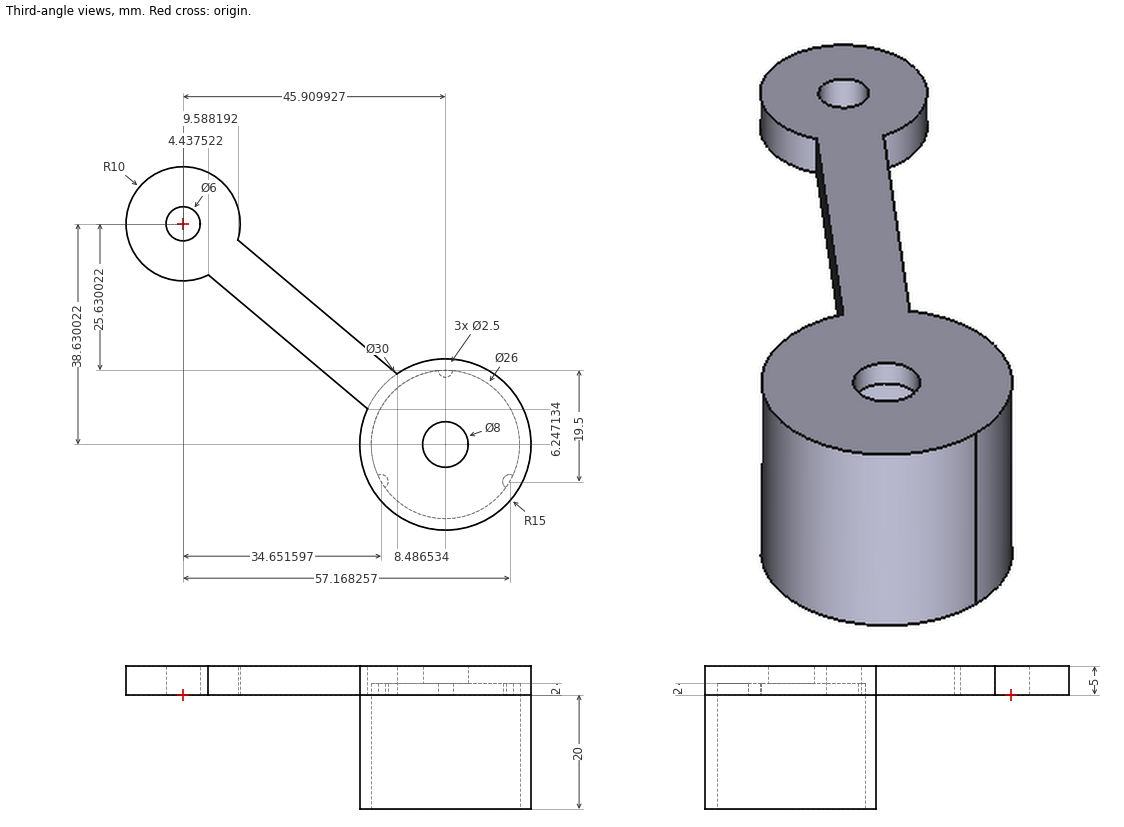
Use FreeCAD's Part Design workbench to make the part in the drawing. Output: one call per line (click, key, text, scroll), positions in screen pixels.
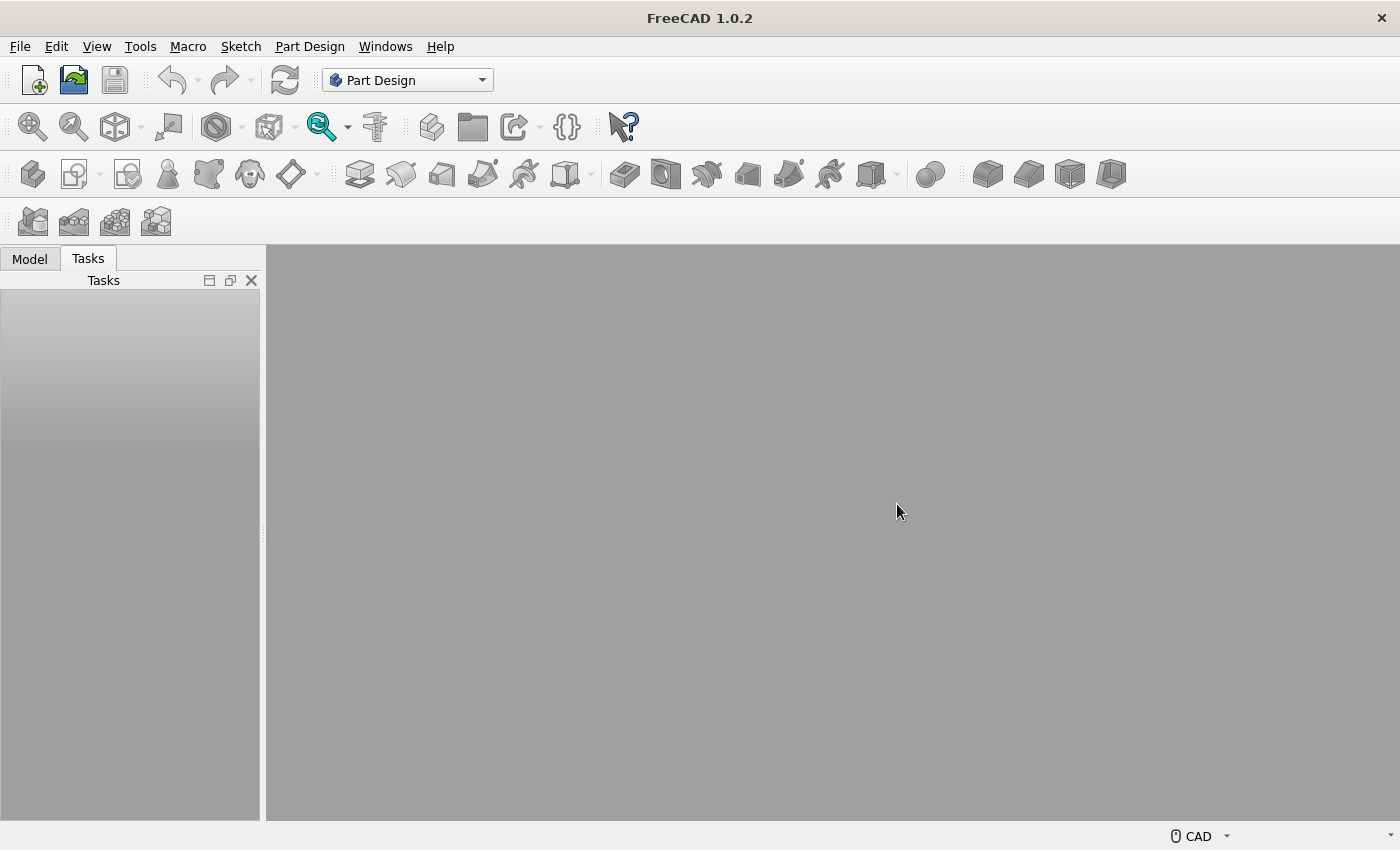
click(33, 80)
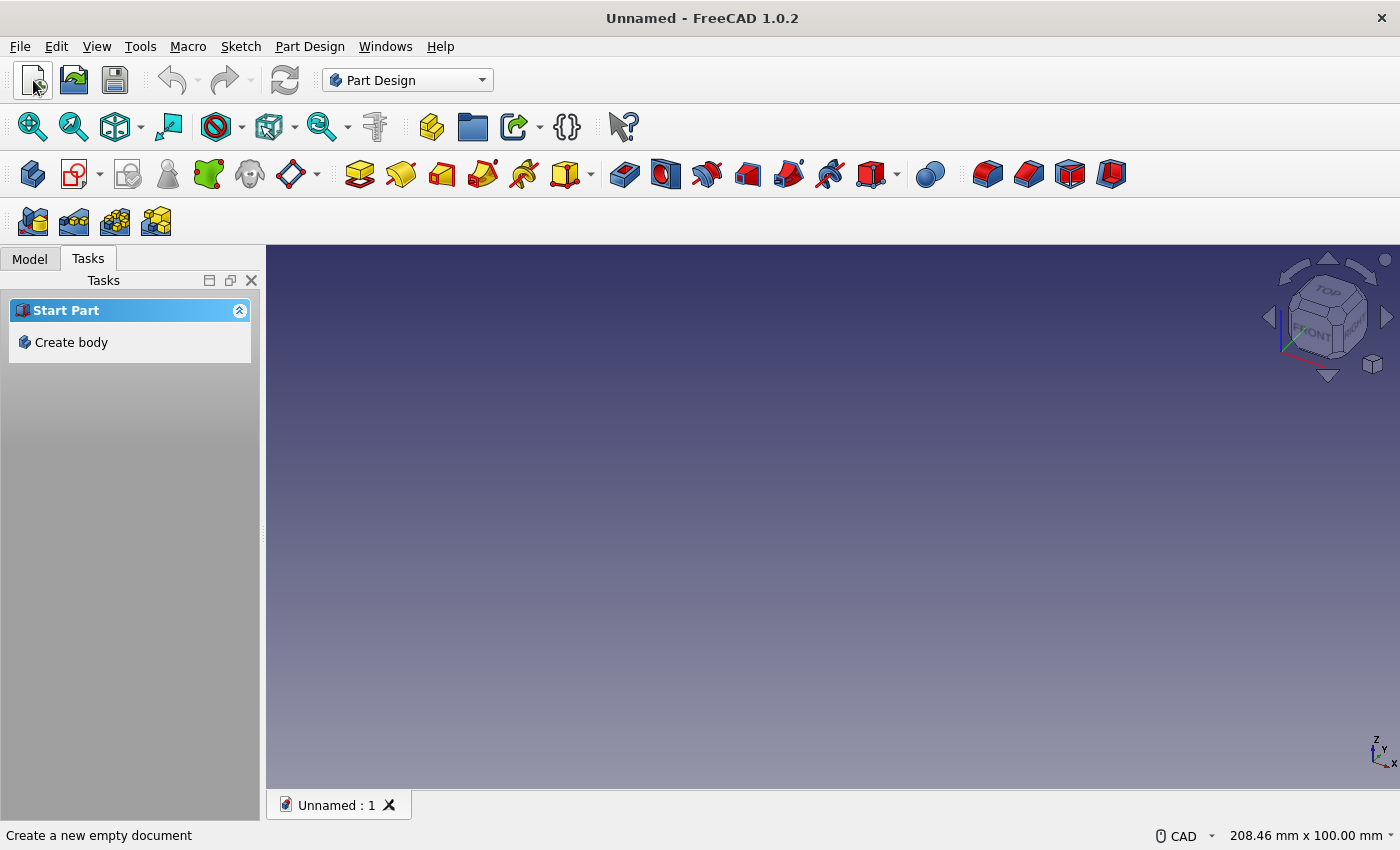
click(74, 174)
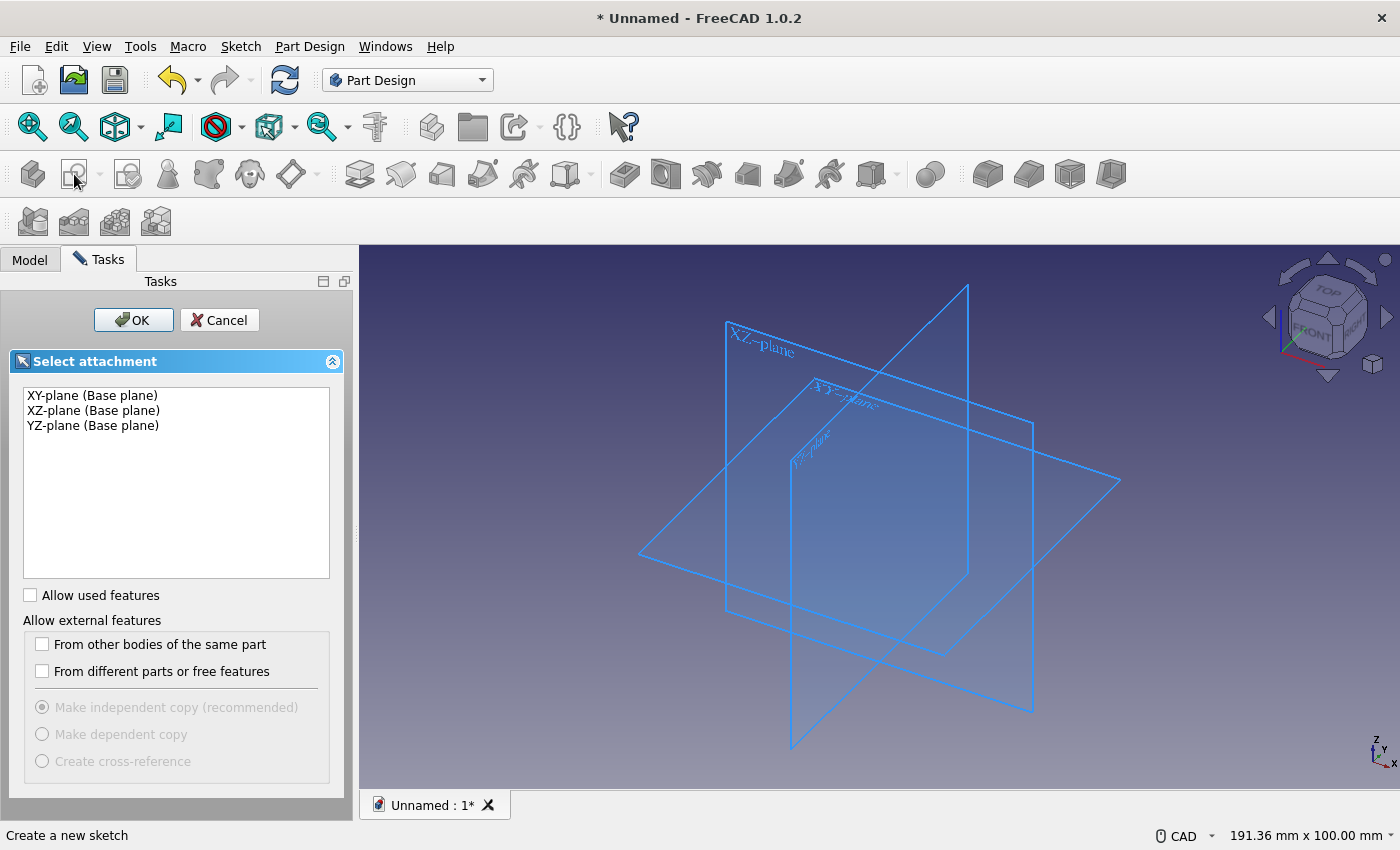
click(84, 396)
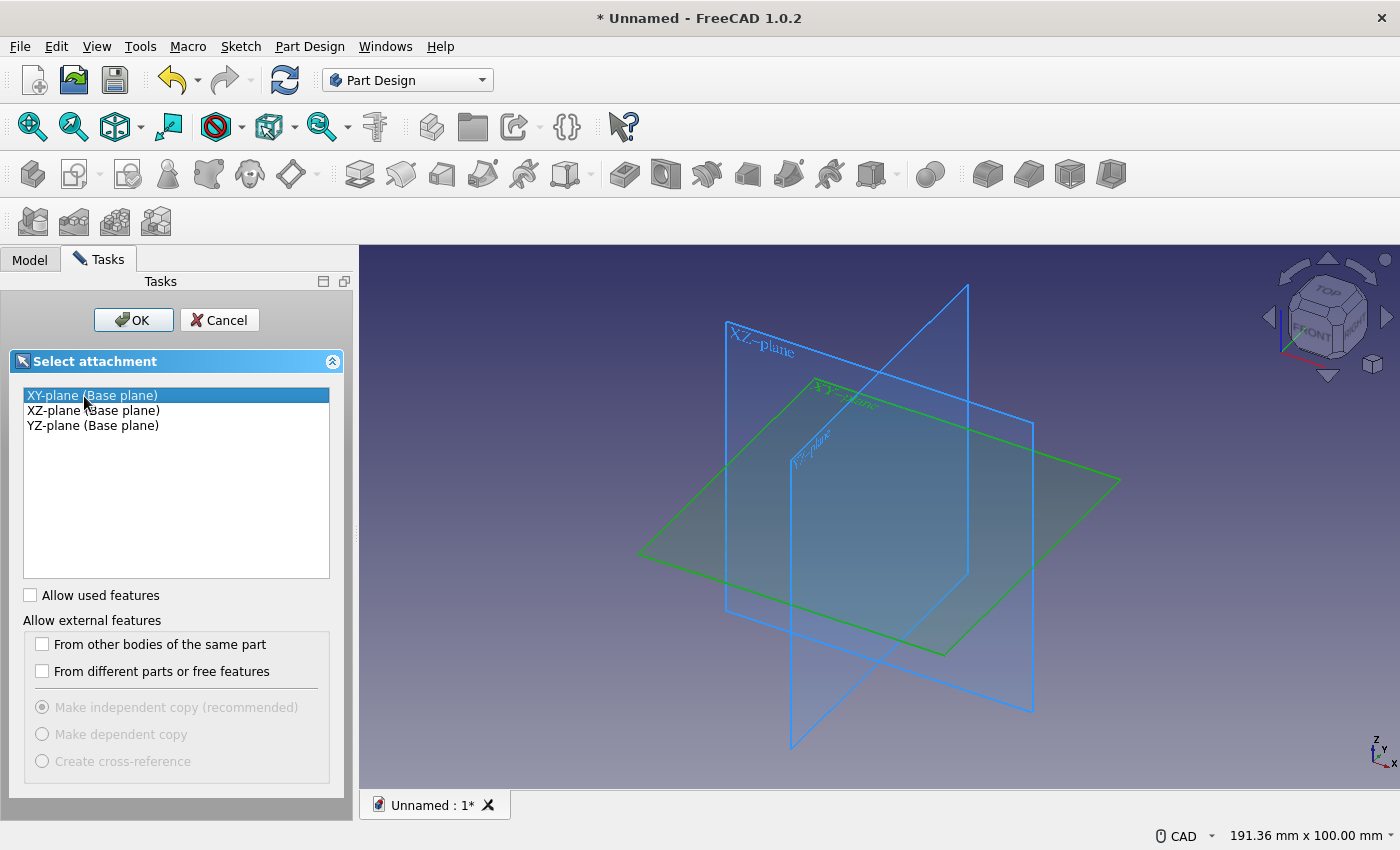
click(134, 320)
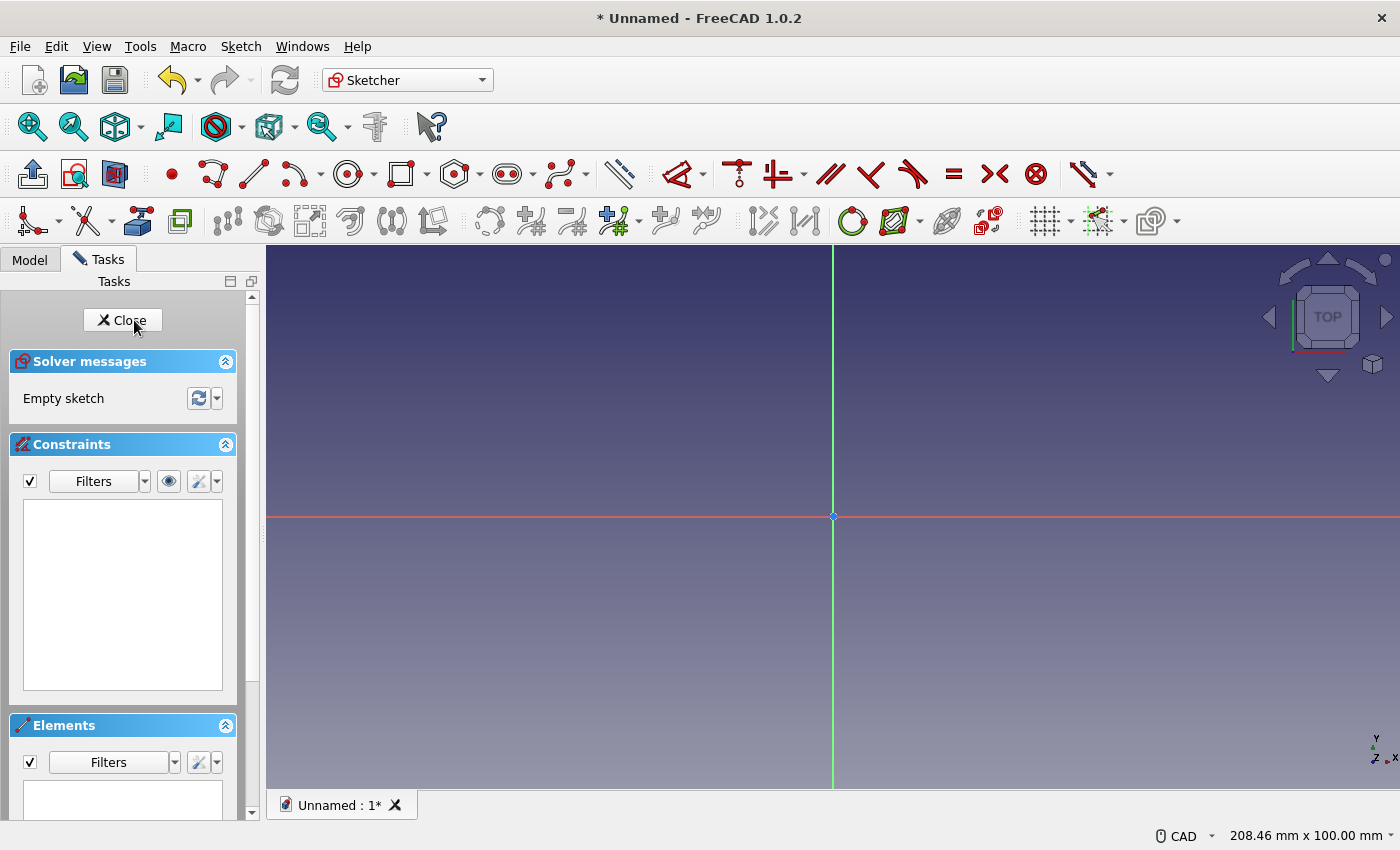
scroll(294, 273, down, 1)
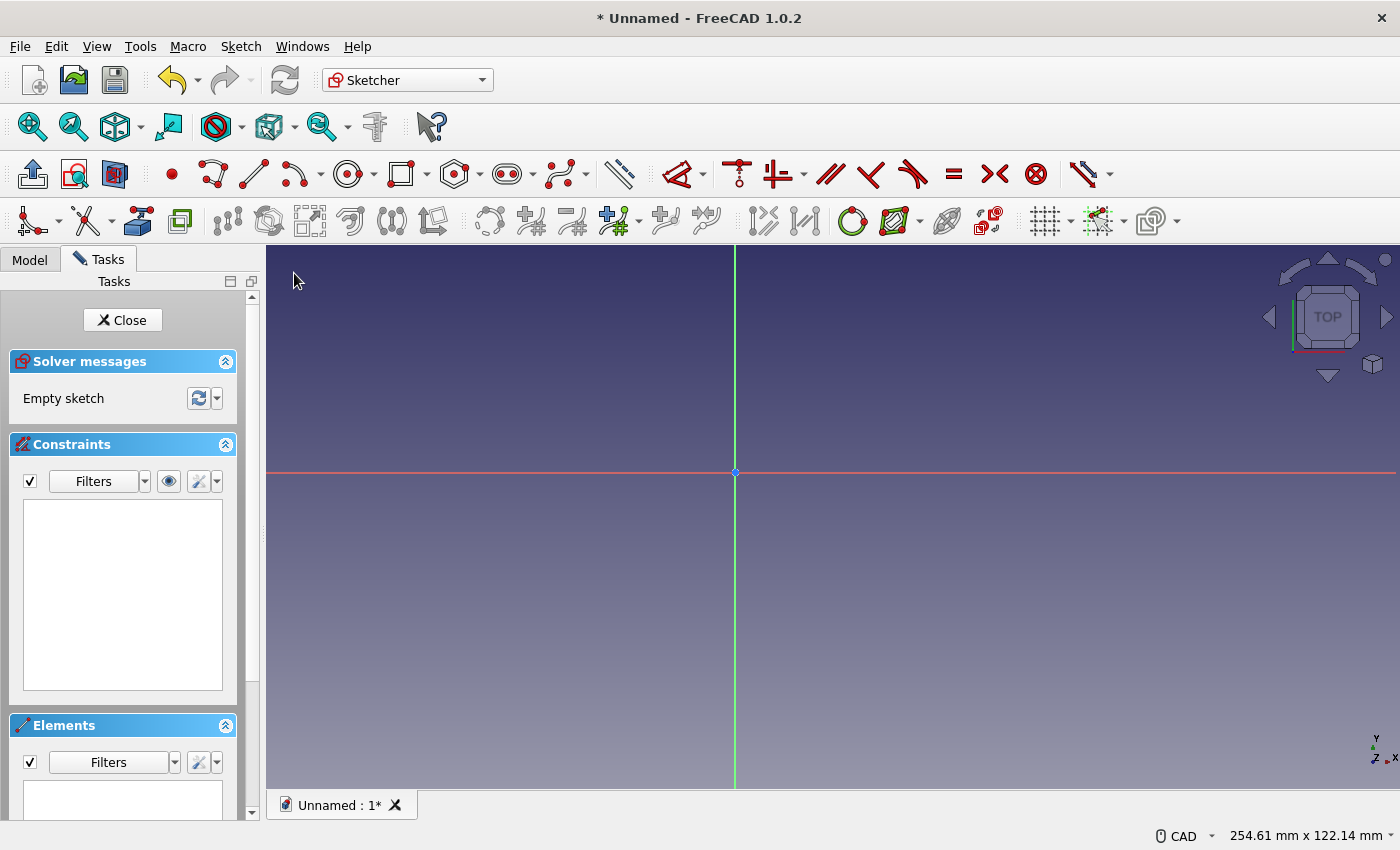
scroll(1012, 666, up, 2)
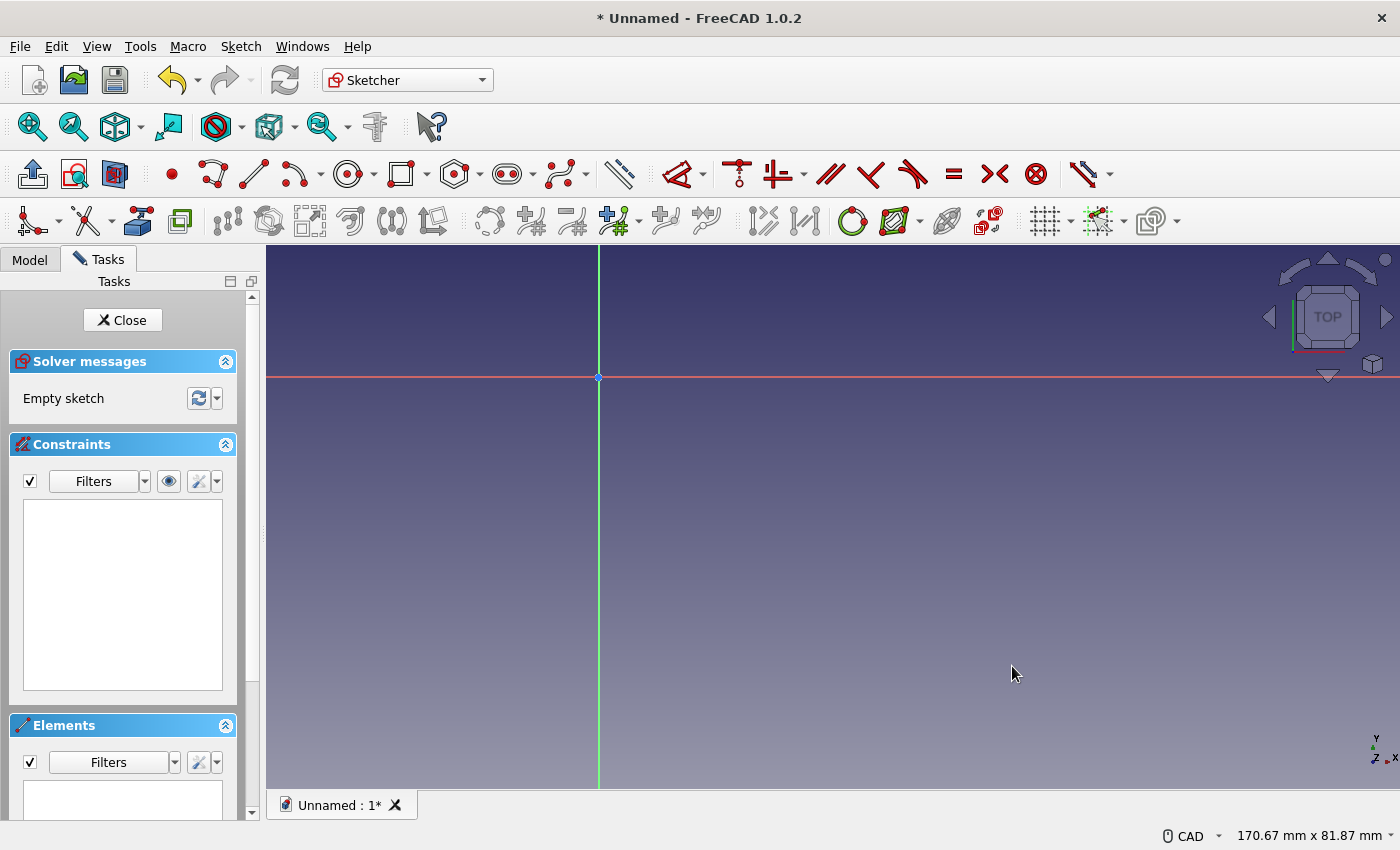
click(254, 174)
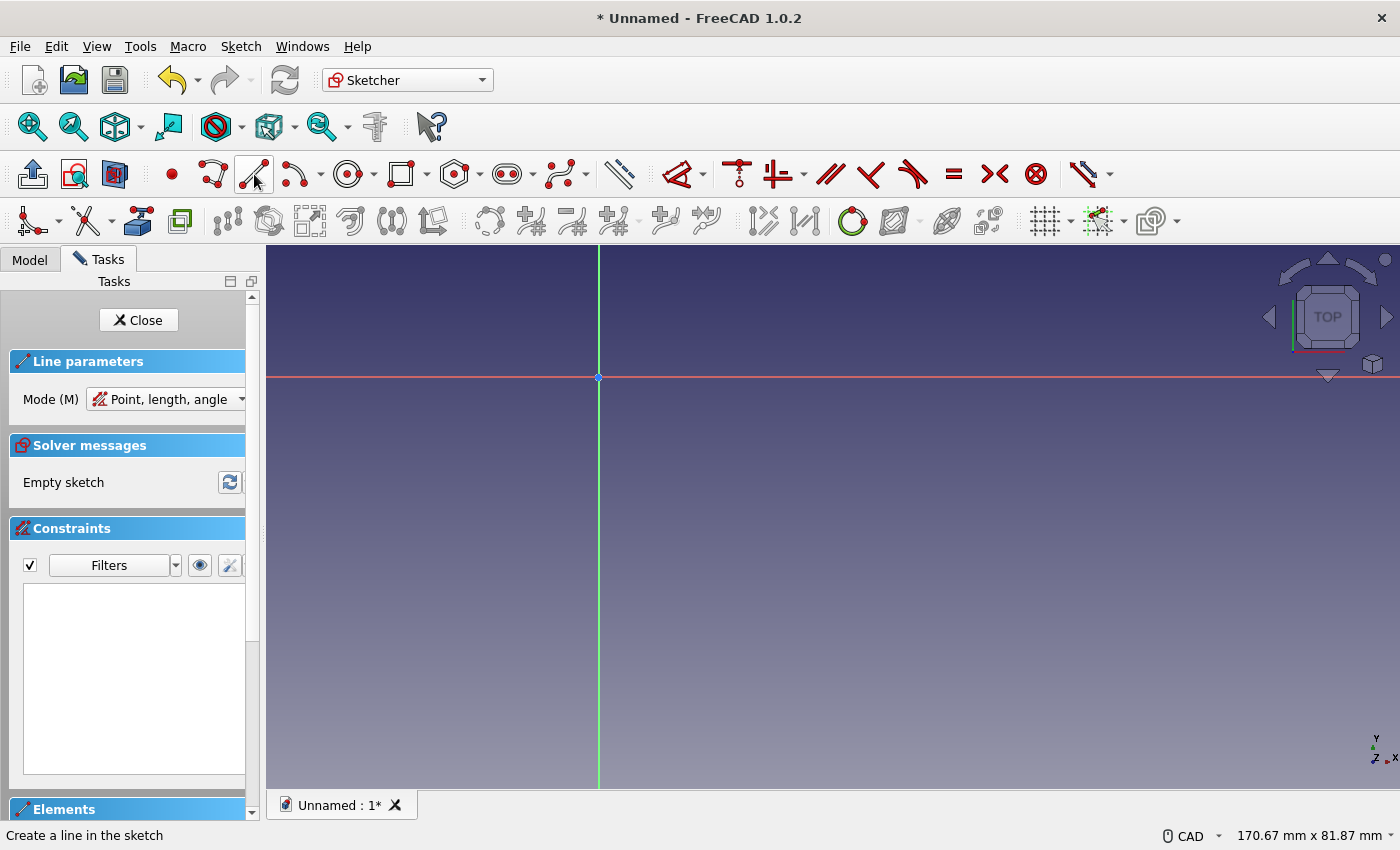
click(628, 437)
click(813, 593)